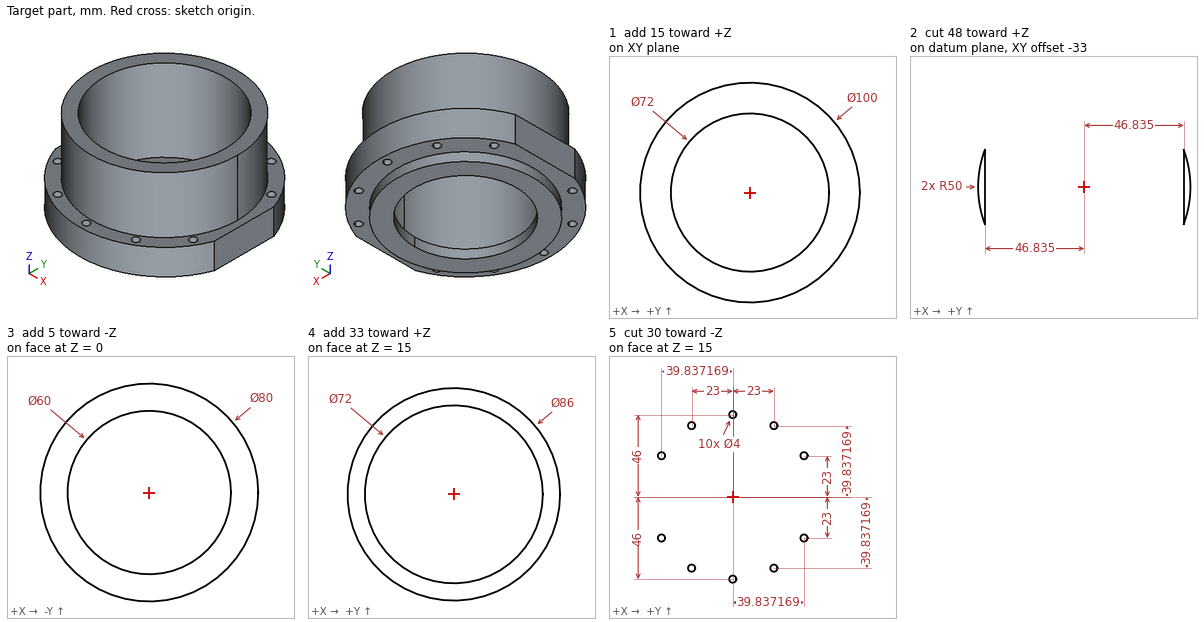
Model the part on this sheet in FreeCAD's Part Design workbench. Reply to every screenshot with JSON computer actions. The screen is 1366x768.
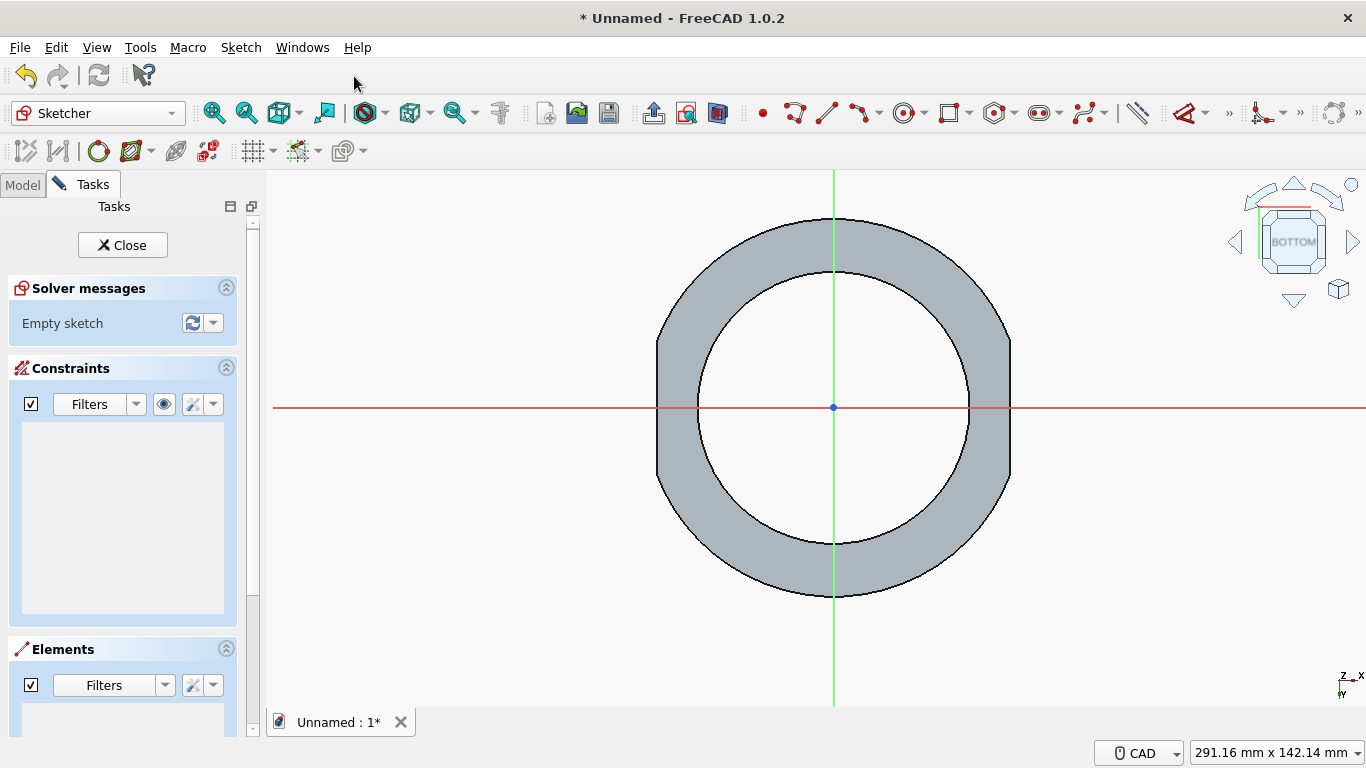
{"action": "left_click", "coordinate": [904, 114]}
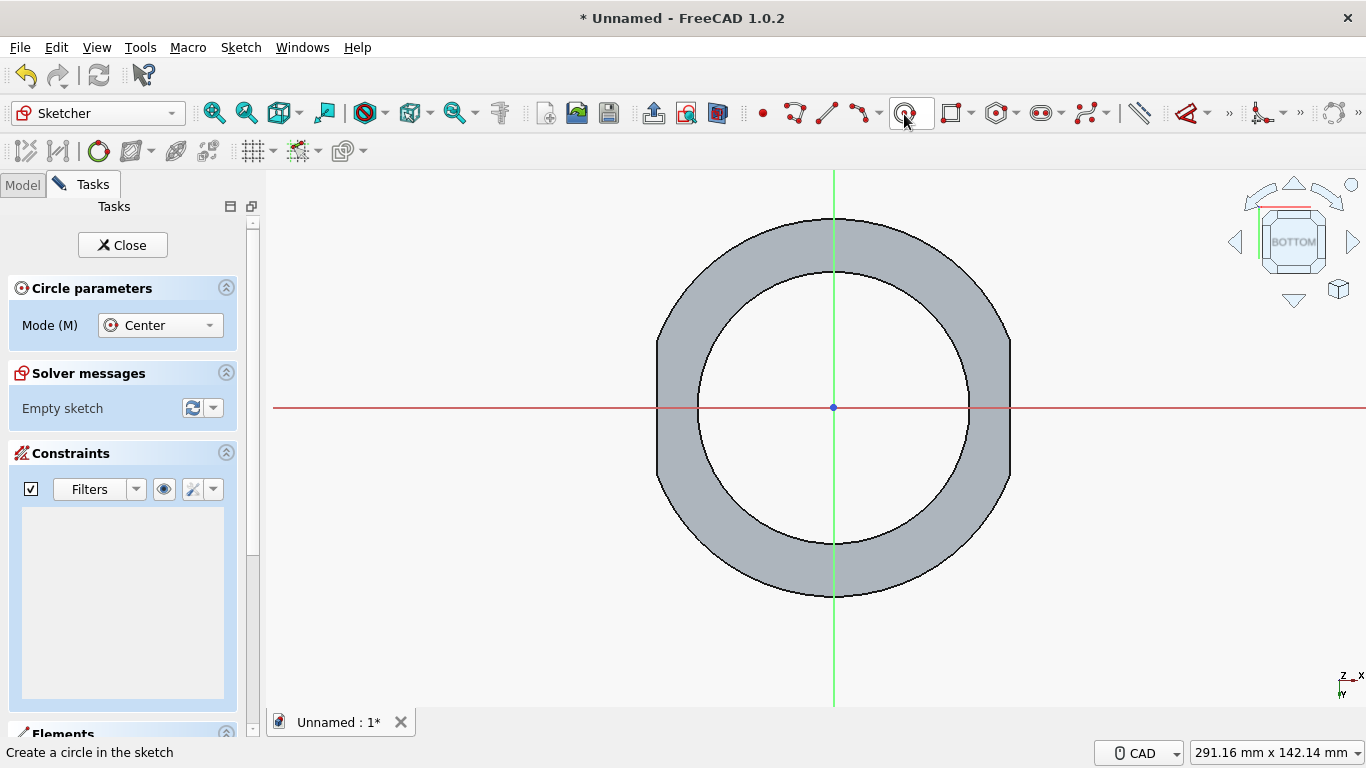
{"action": "left_click", "coordinate": [834, 408]}
{"action": "mouse_move", "coordinate": [940, 301]}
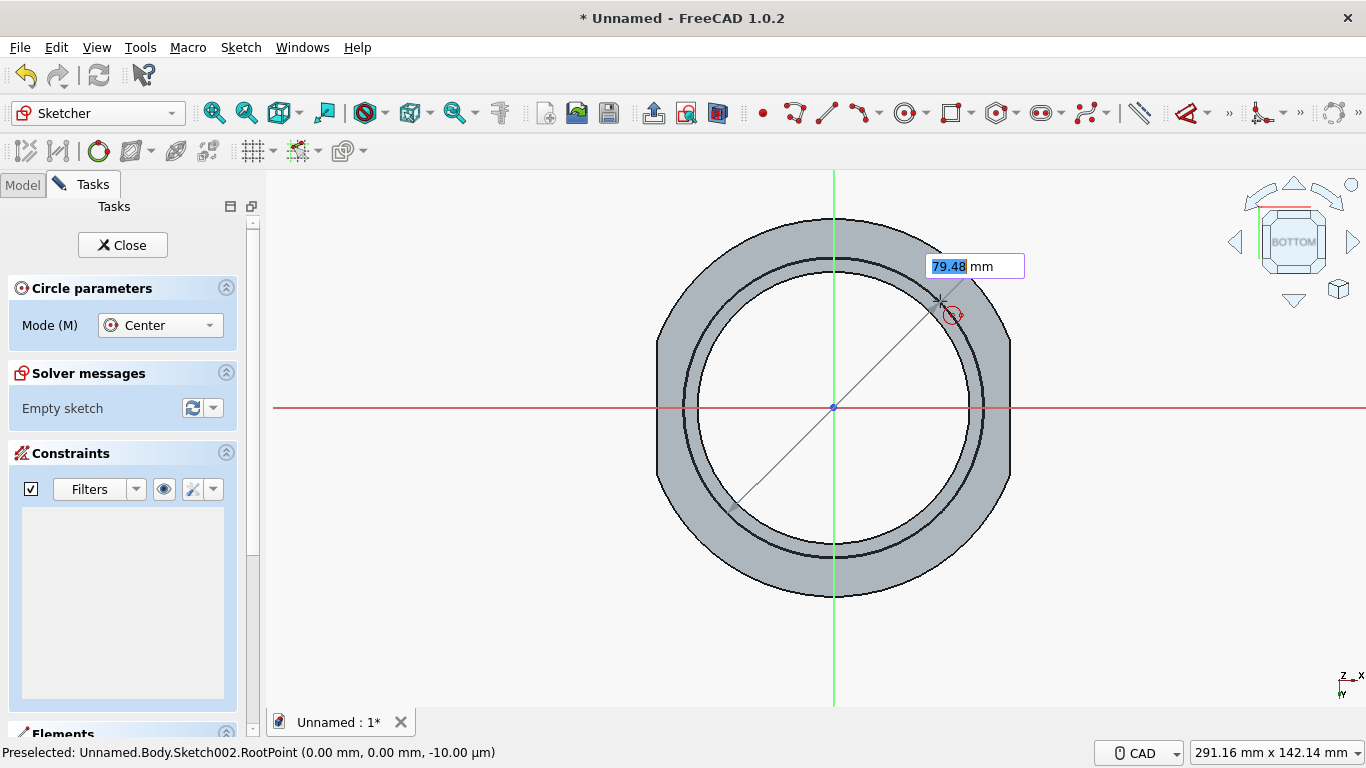
{"action": "type", "text": "80"}
{"action": "key", "text": "Return"}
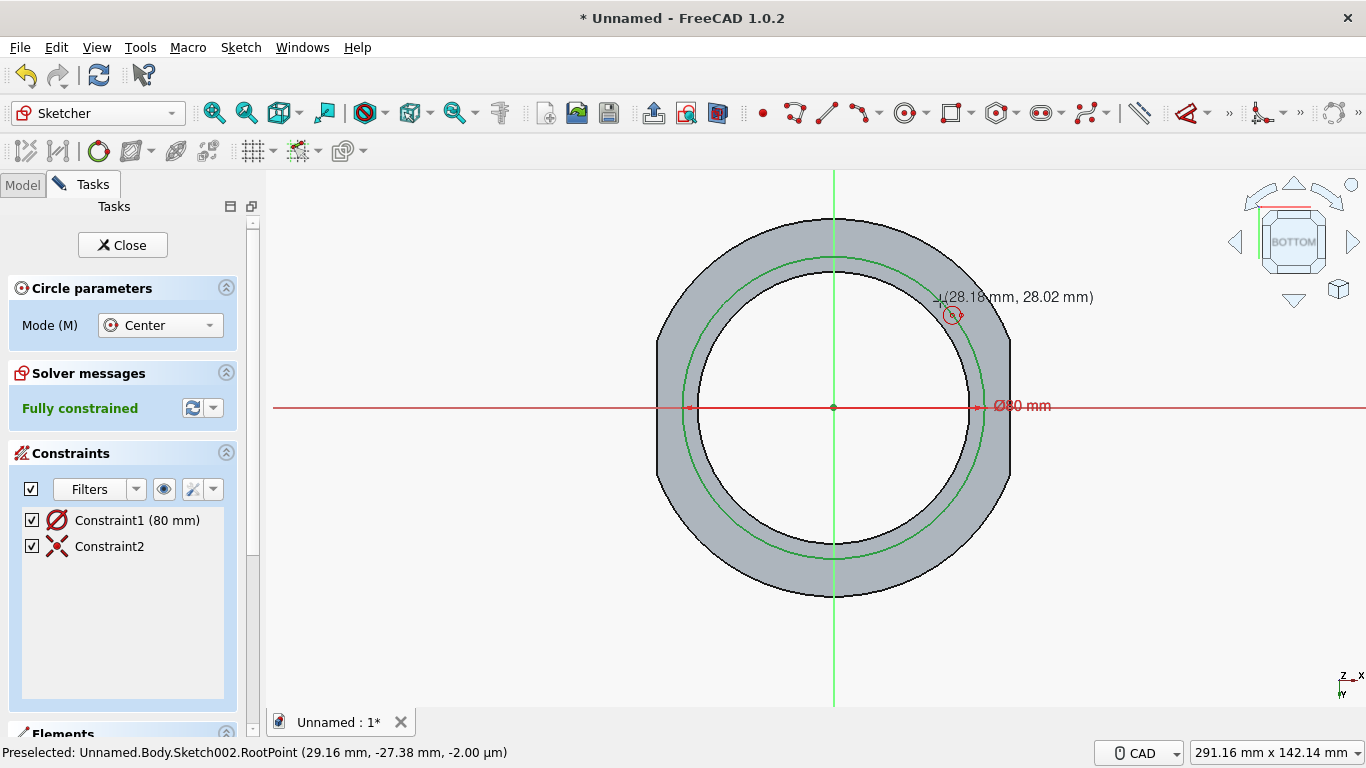
{"action": "left_click", "coordinate": [834, 408]}
{"action": "mouse_move", "coordinate": [914, 328]}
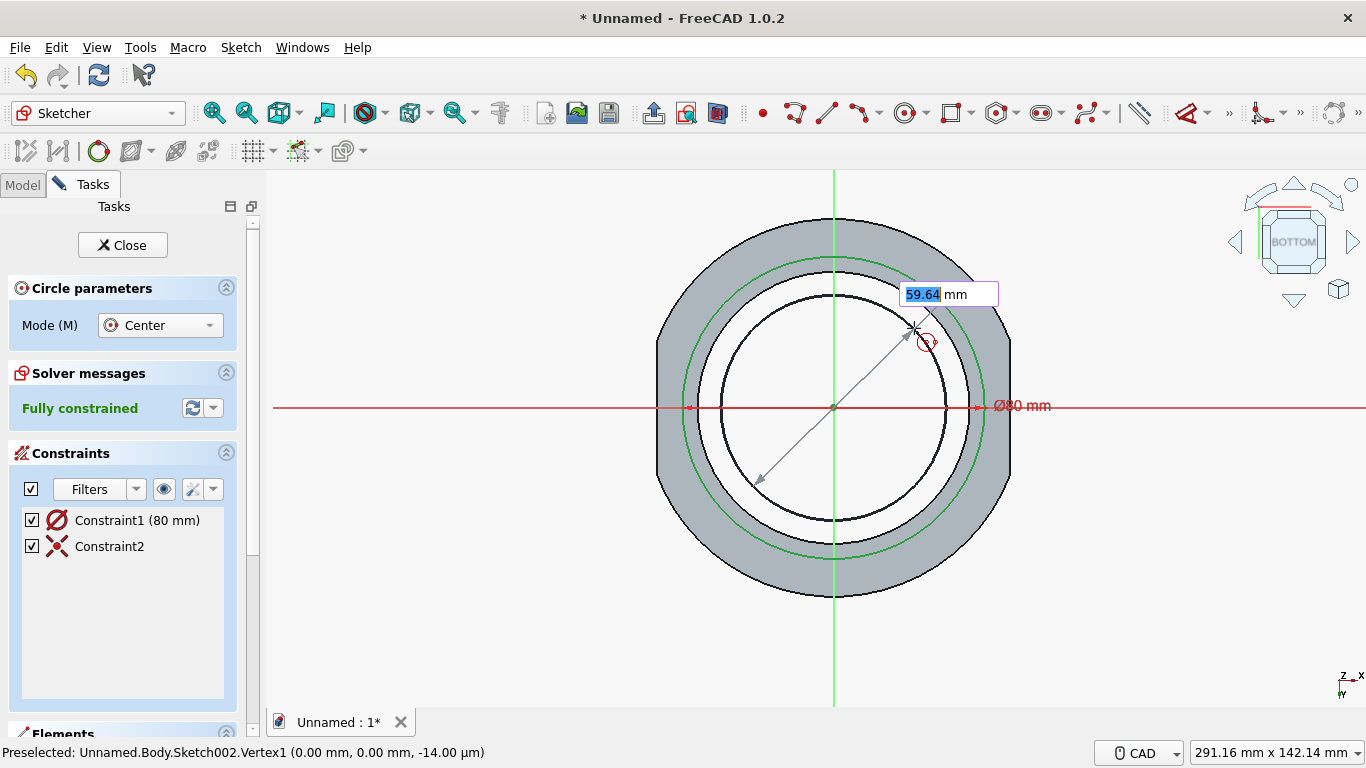
{"action": "type", "text": "60"}
{"action": "key", "text": "Return"}
{"action": "key", "text": "Escape"}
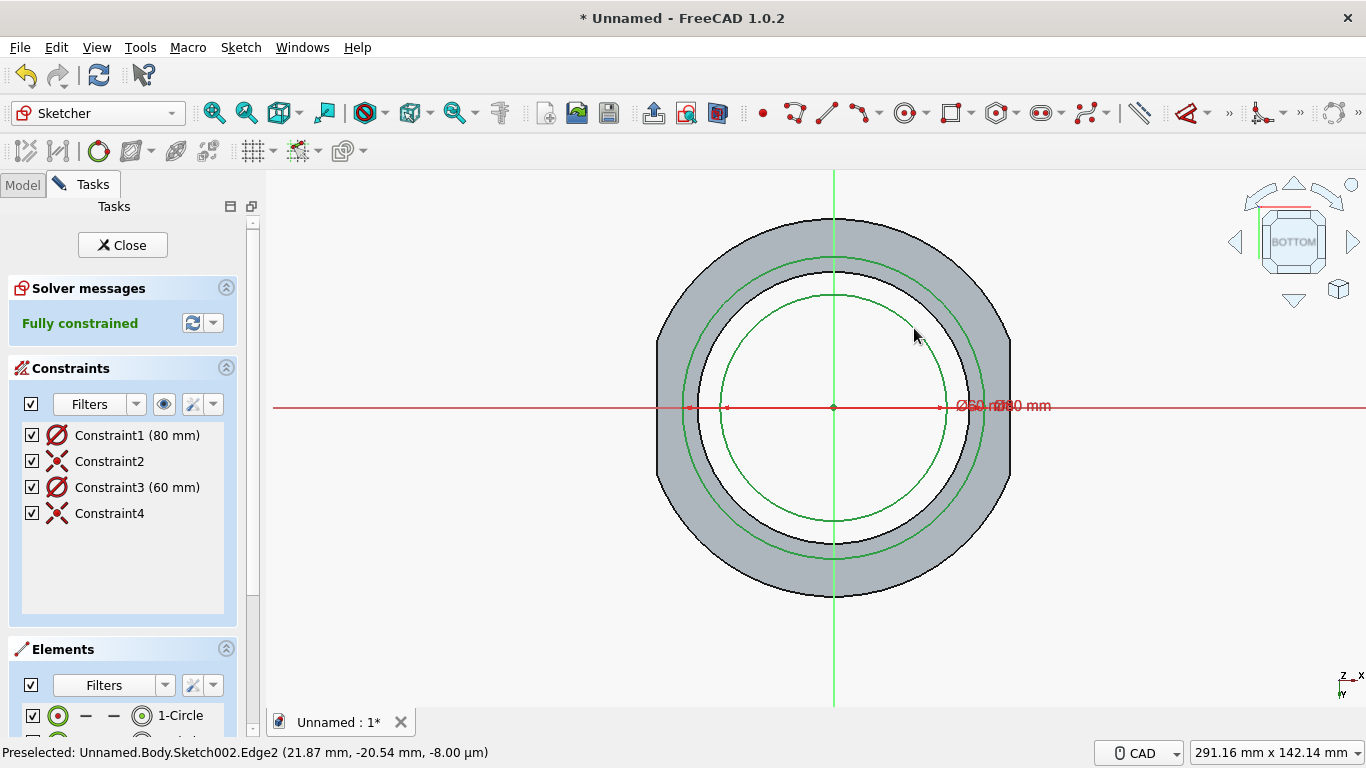
{"action": "left_click", "coordinate": [123, 245]}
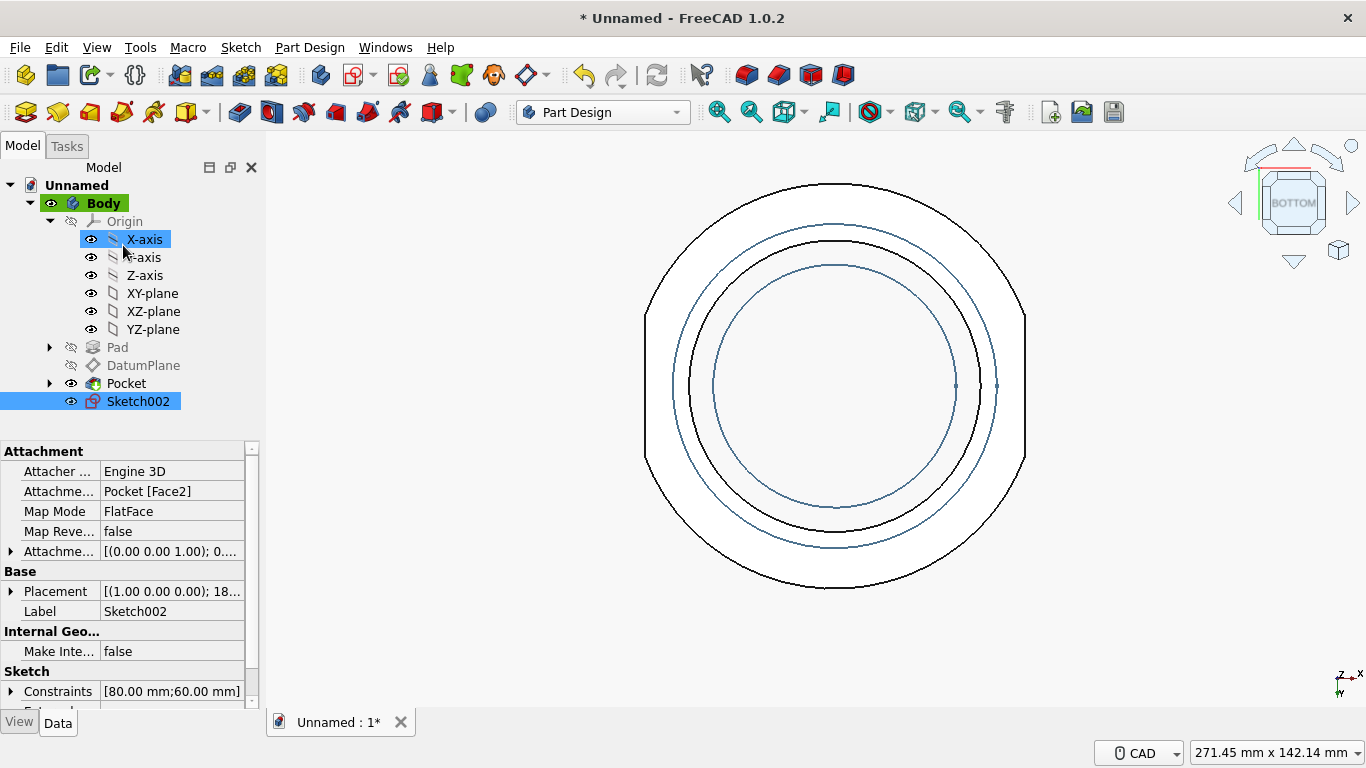
{"action": "left_click", "coordinate": [26, 112]}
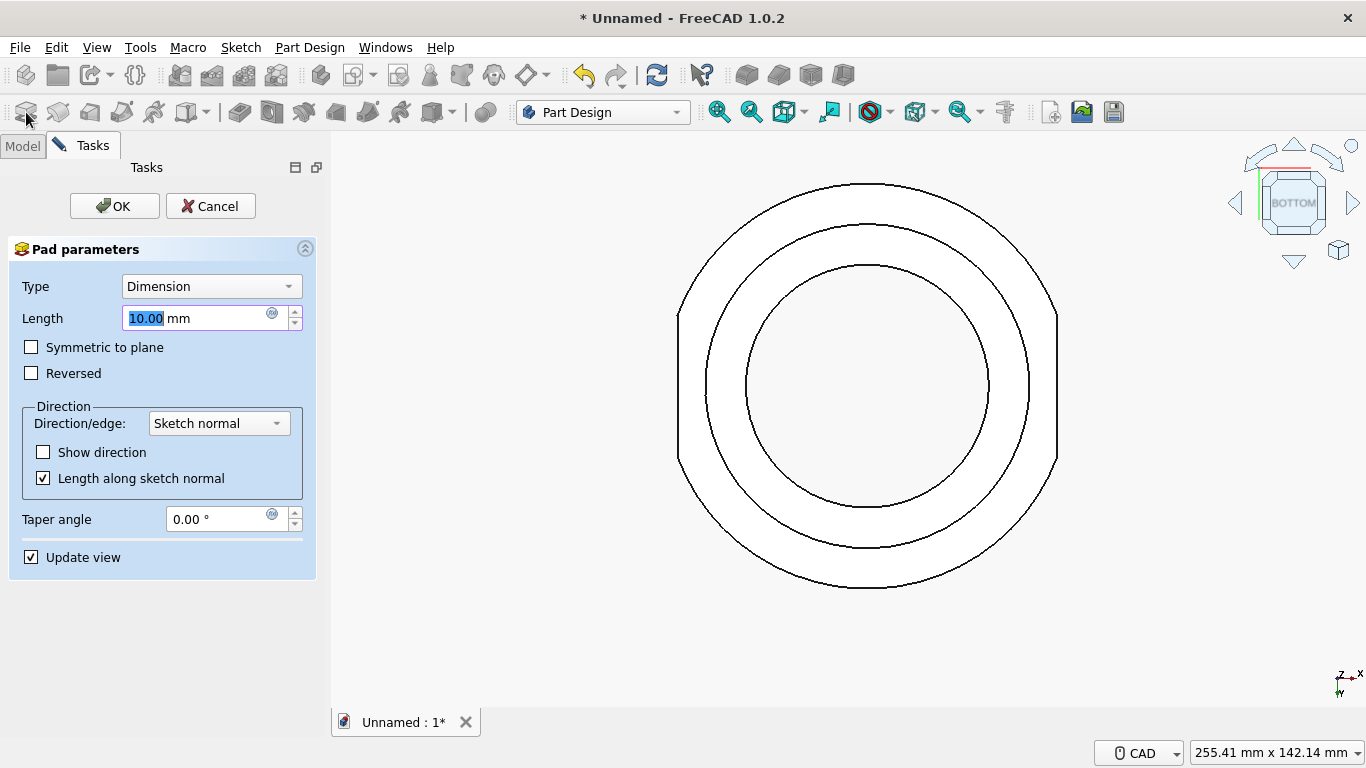
{"action": "type", "text": "5"}
{"action": "key", "text": "Tab"}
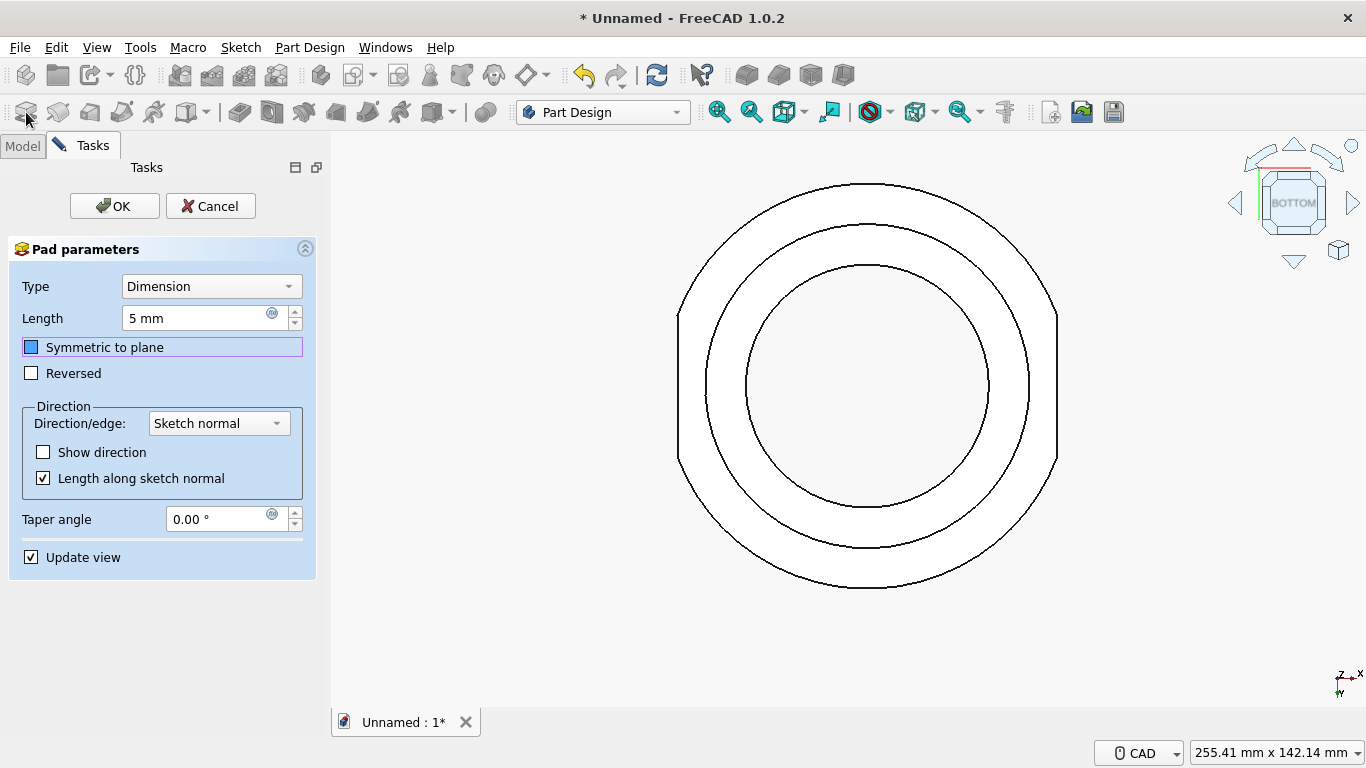
{"action": "left_click", "coordinate": [115, 206]}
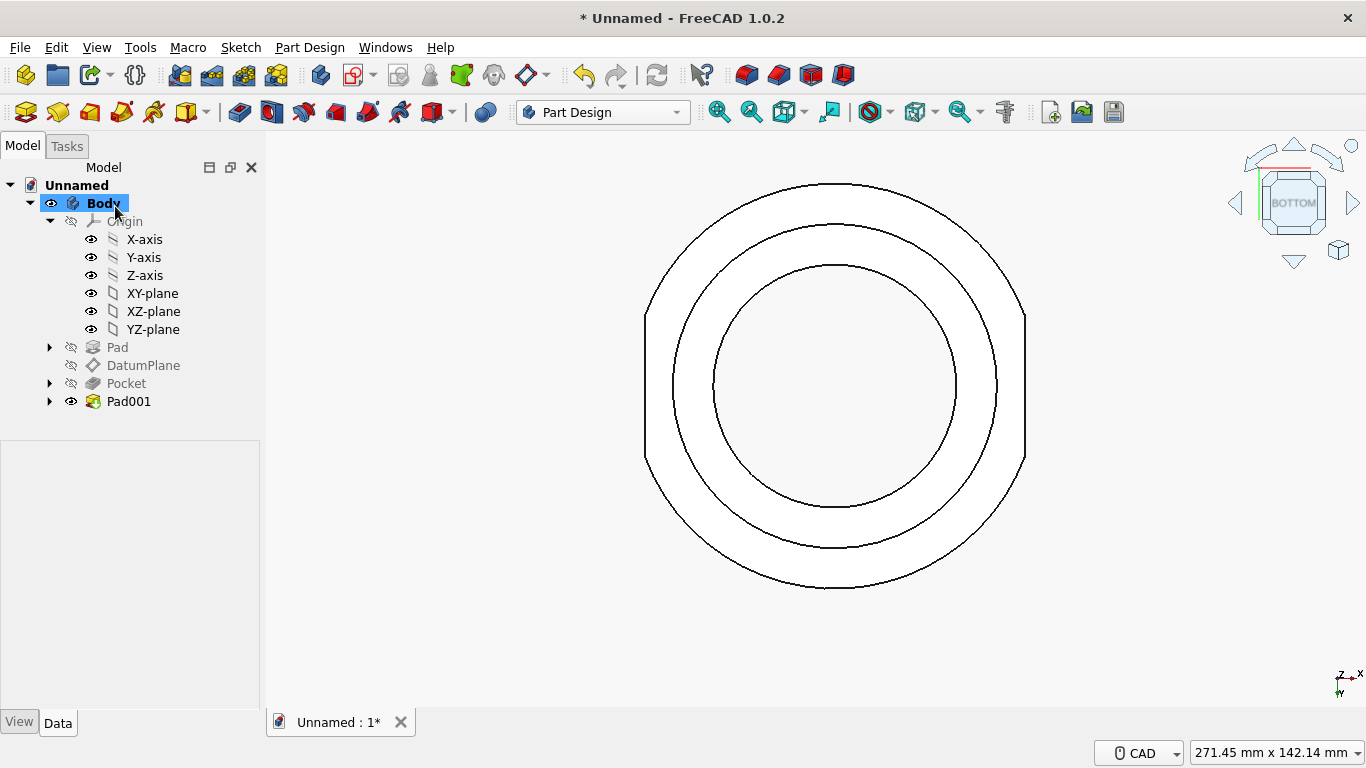
{"action": "key", "text": "0"}